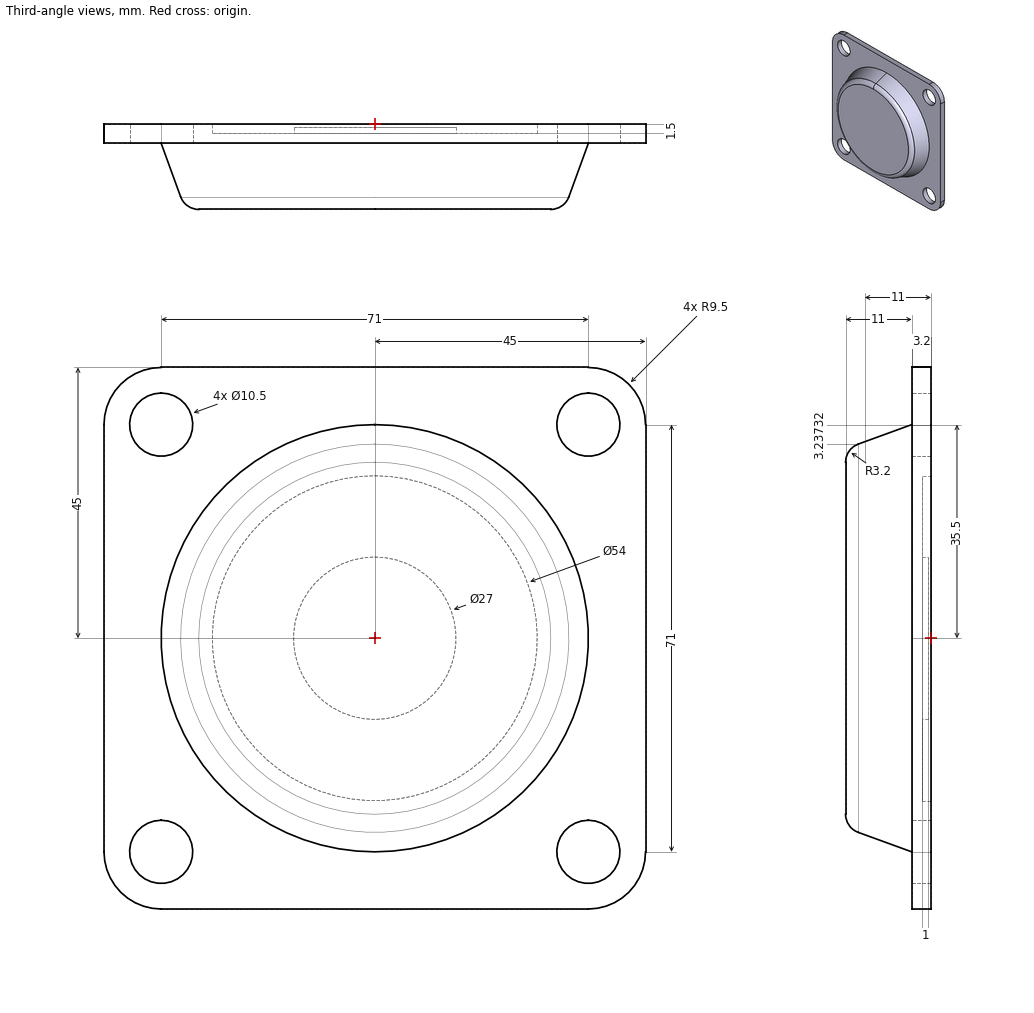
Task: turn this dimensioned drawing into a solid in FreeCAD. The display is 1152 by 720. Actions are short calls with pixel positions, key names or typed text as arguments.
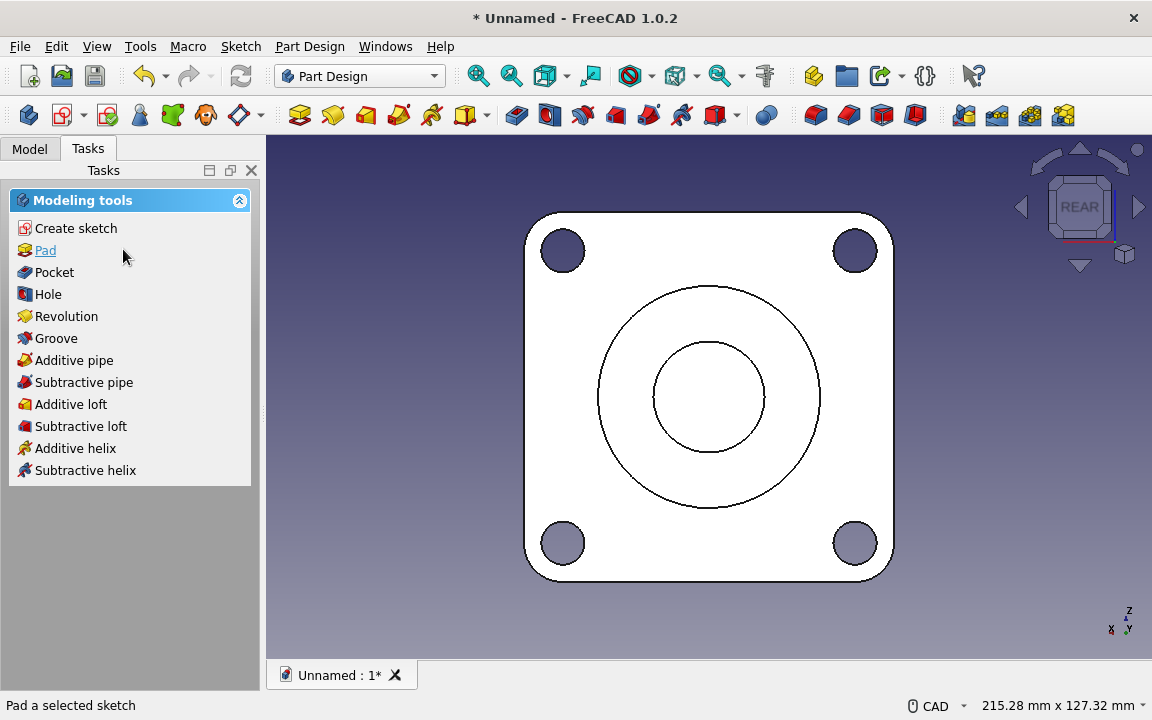
click(333, 116)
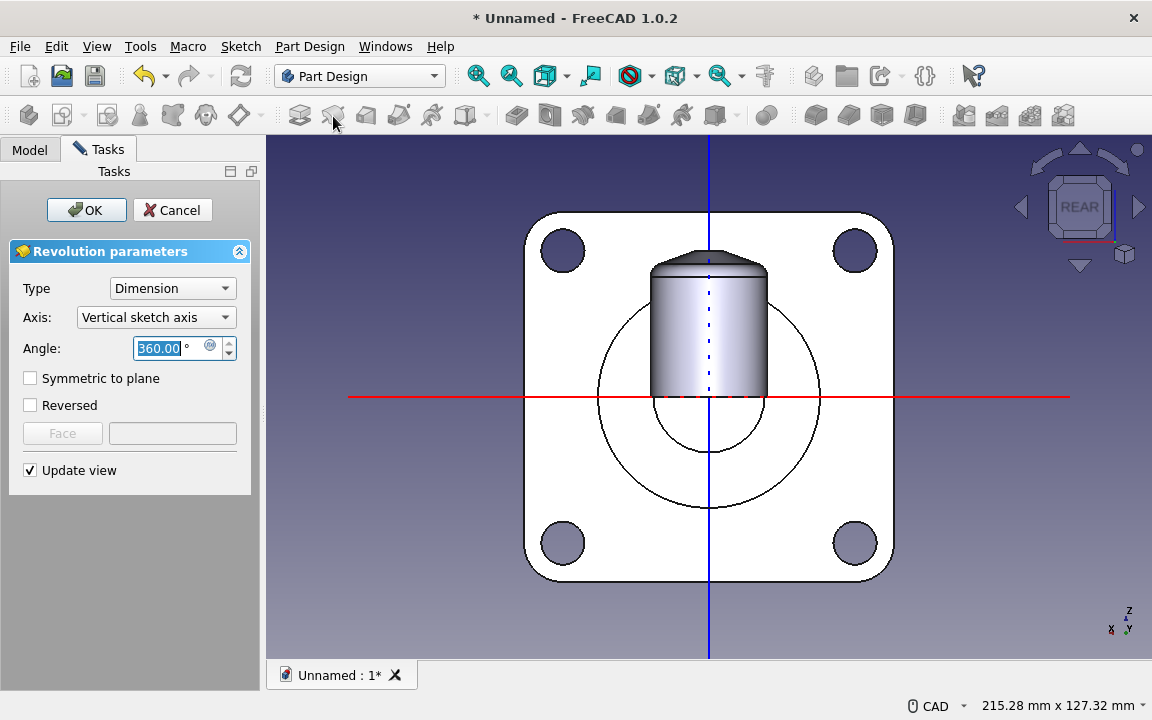
click(157, 318)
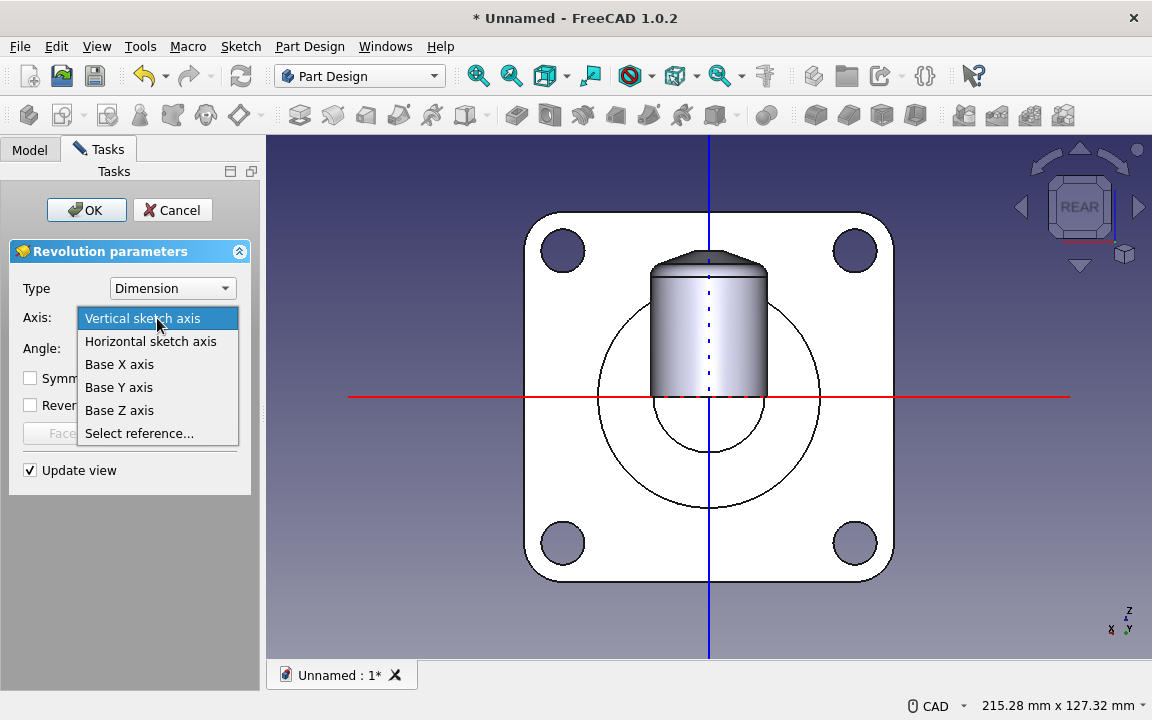
click(156, 342)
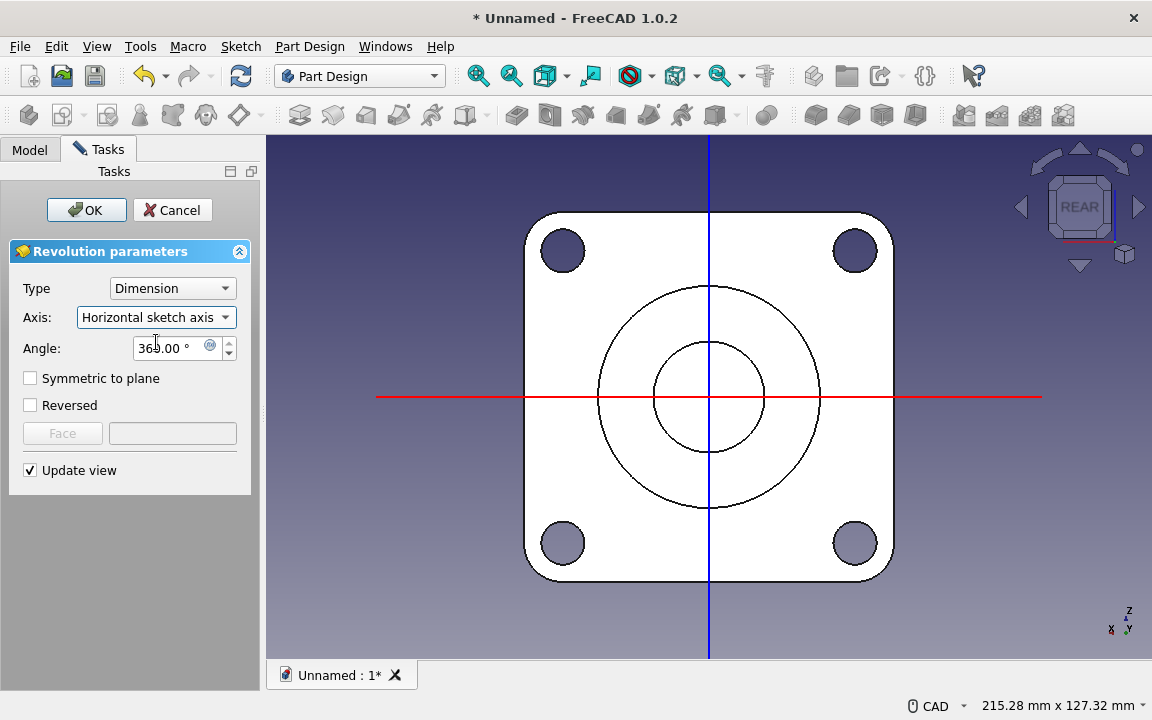
click(87, 210)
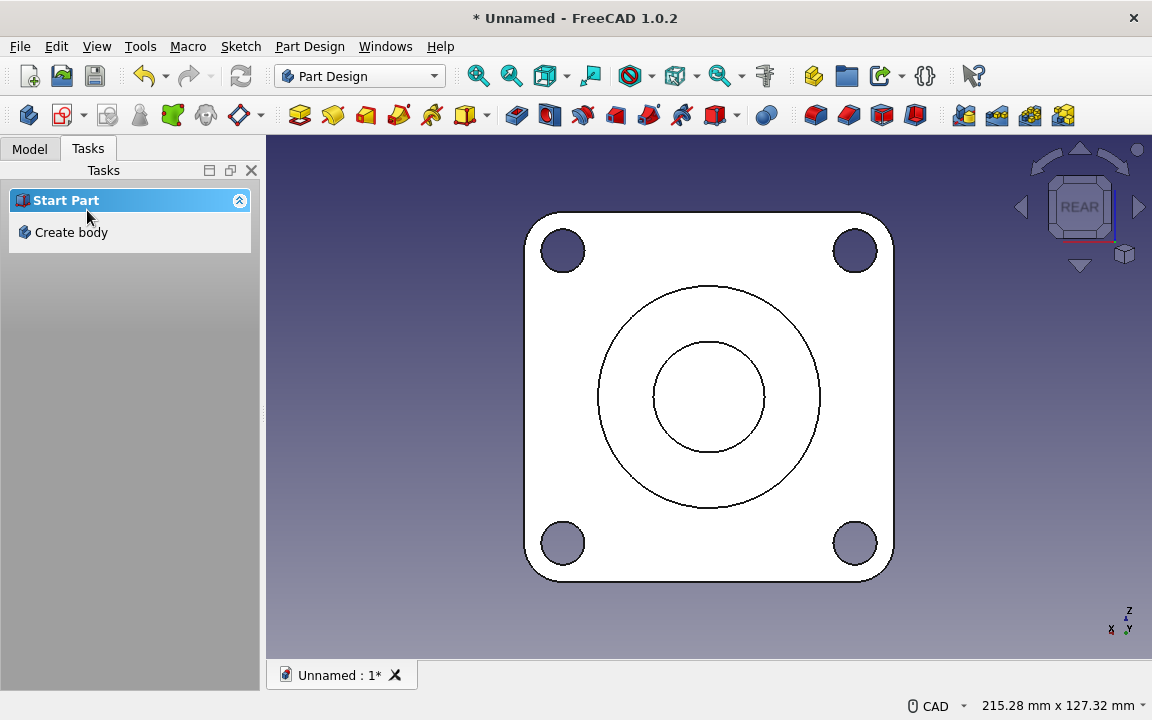
key(0)